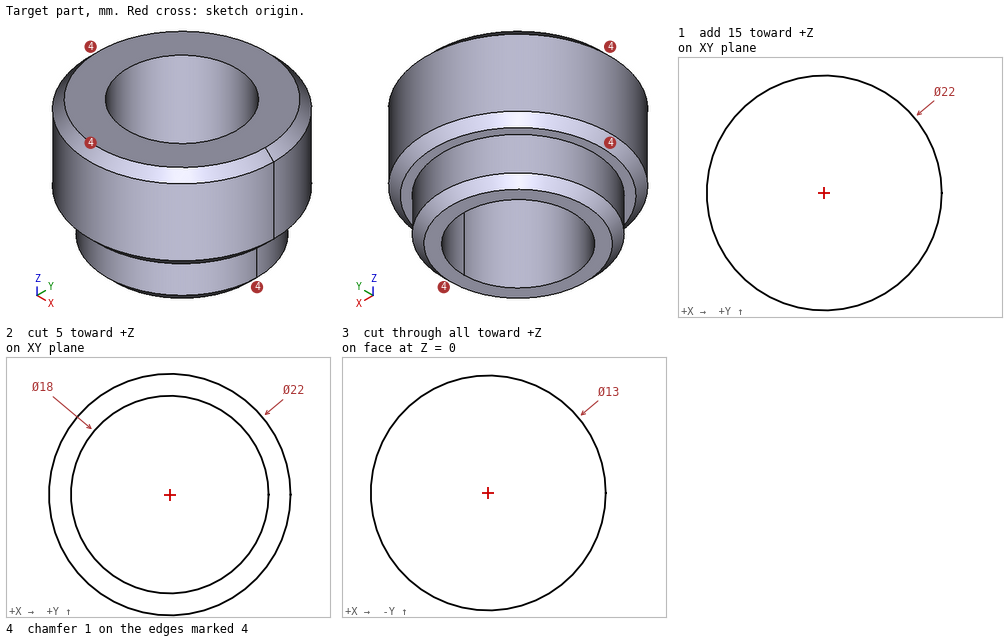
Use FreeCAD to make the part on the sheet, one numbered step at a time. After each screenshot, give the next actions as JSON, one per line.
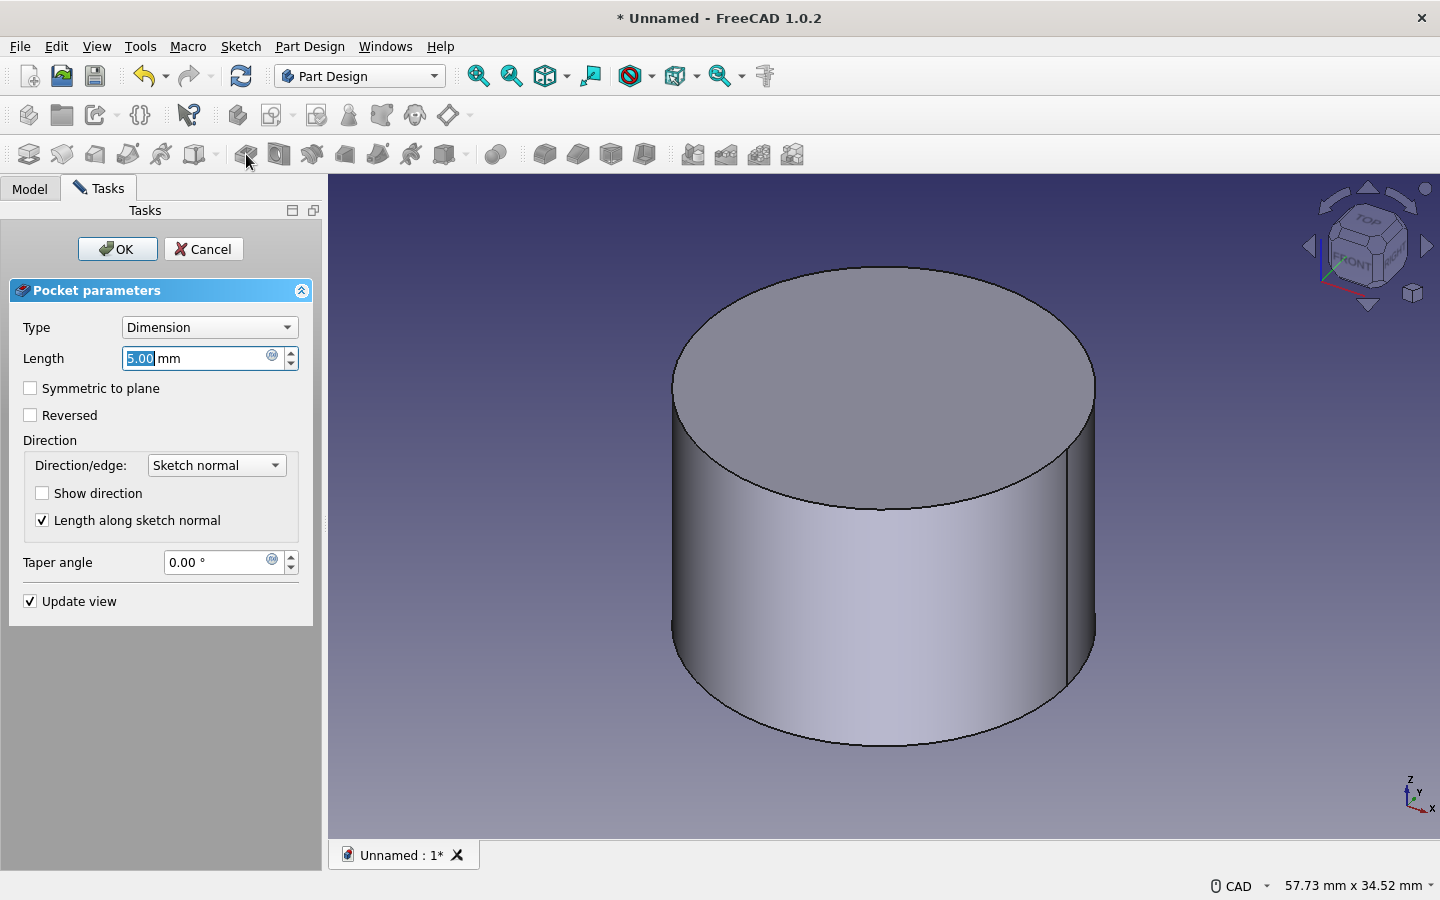
{"action": "type", "text": "5"}
{"action": "key", "text": "Tab"}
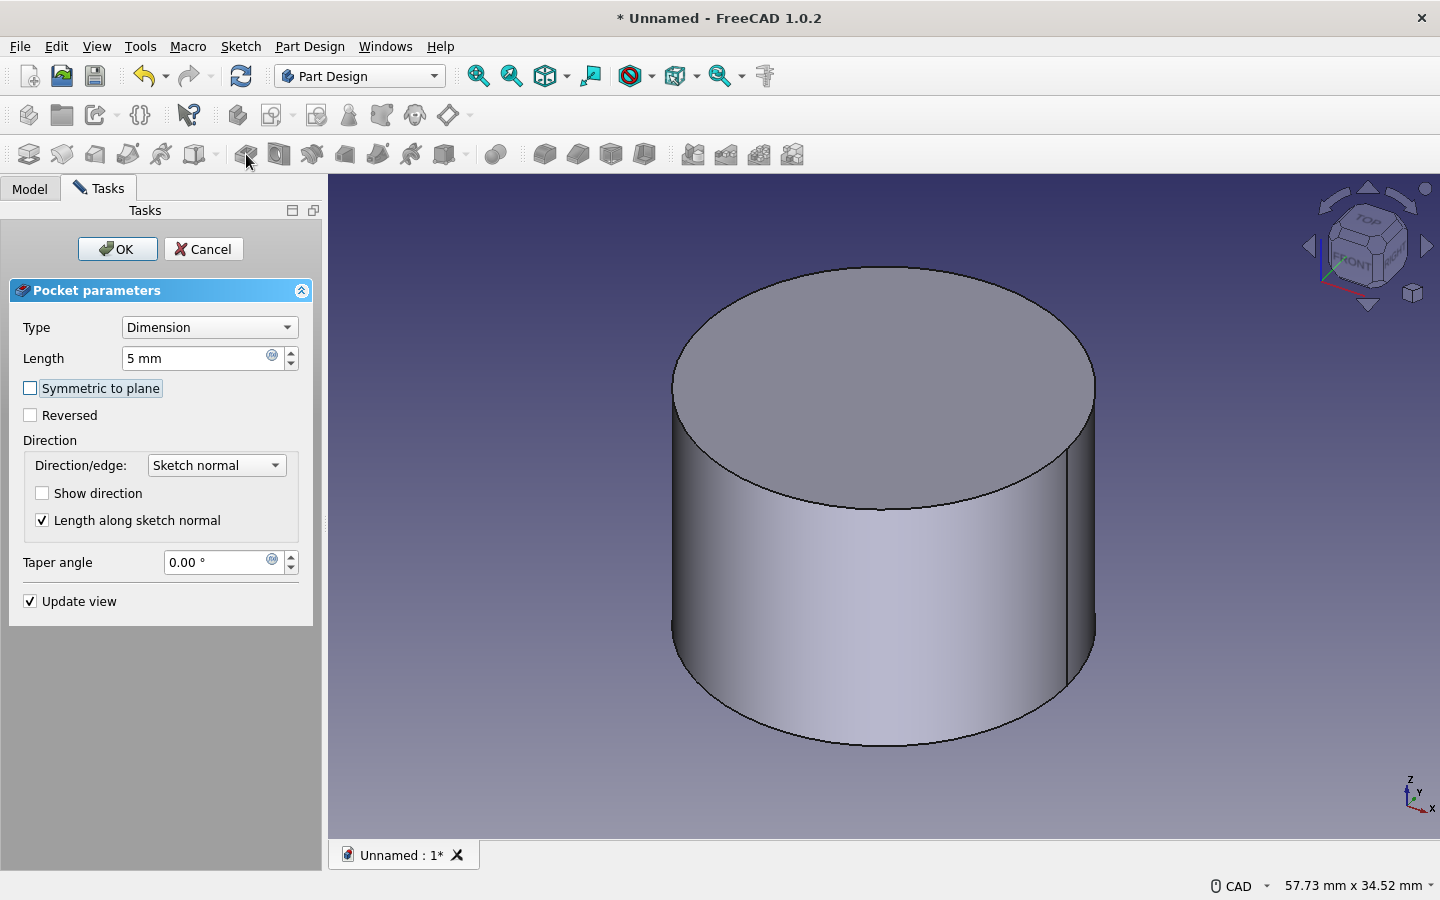
{"action": "left_click", "coordinate": [31, 415]}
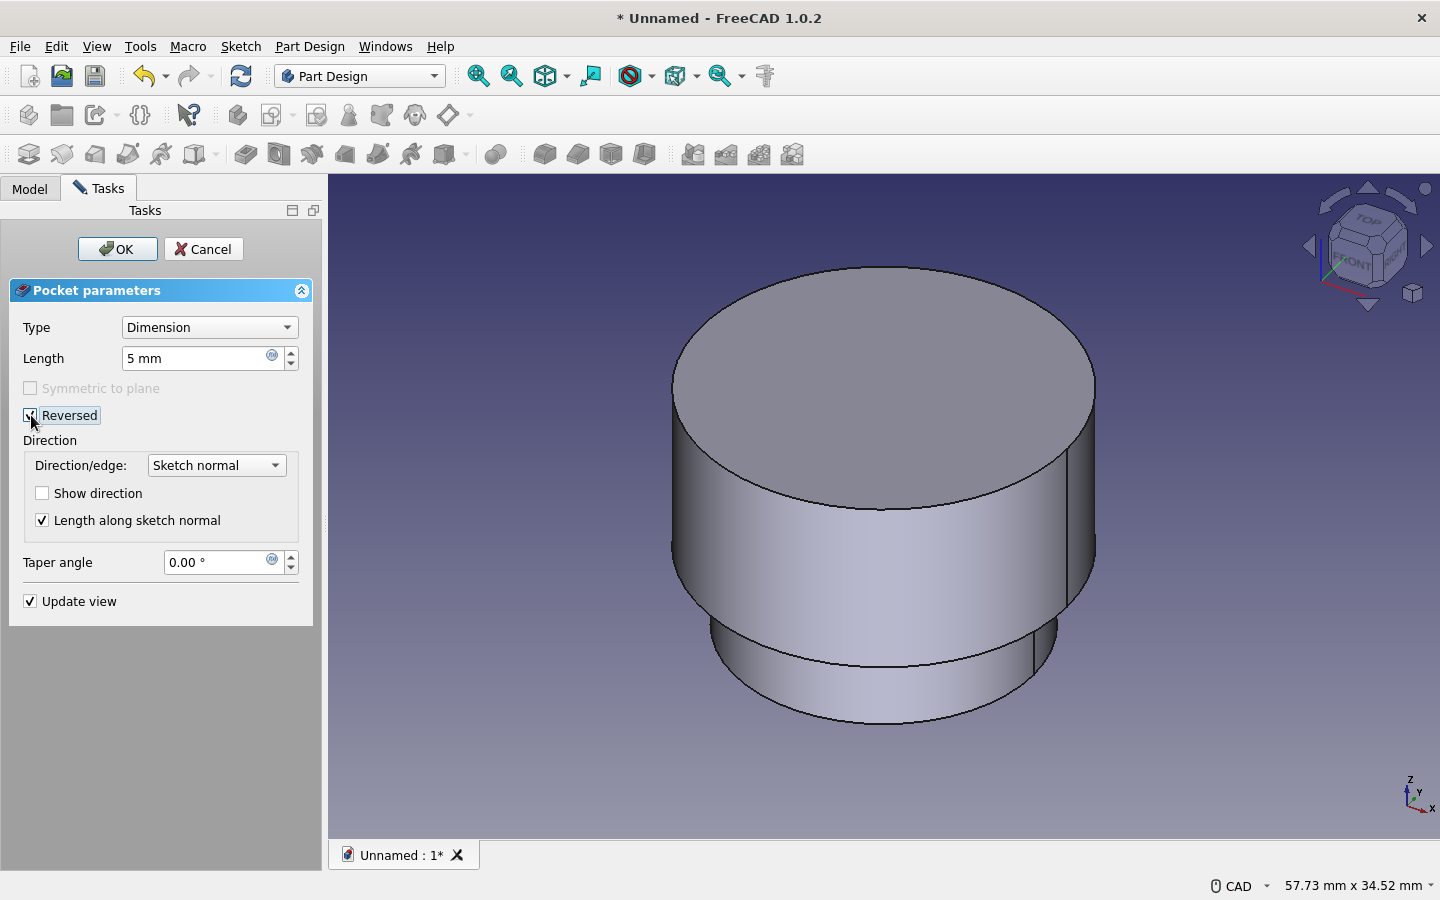
{"action": "left_click", "coordinate": [118, 249]}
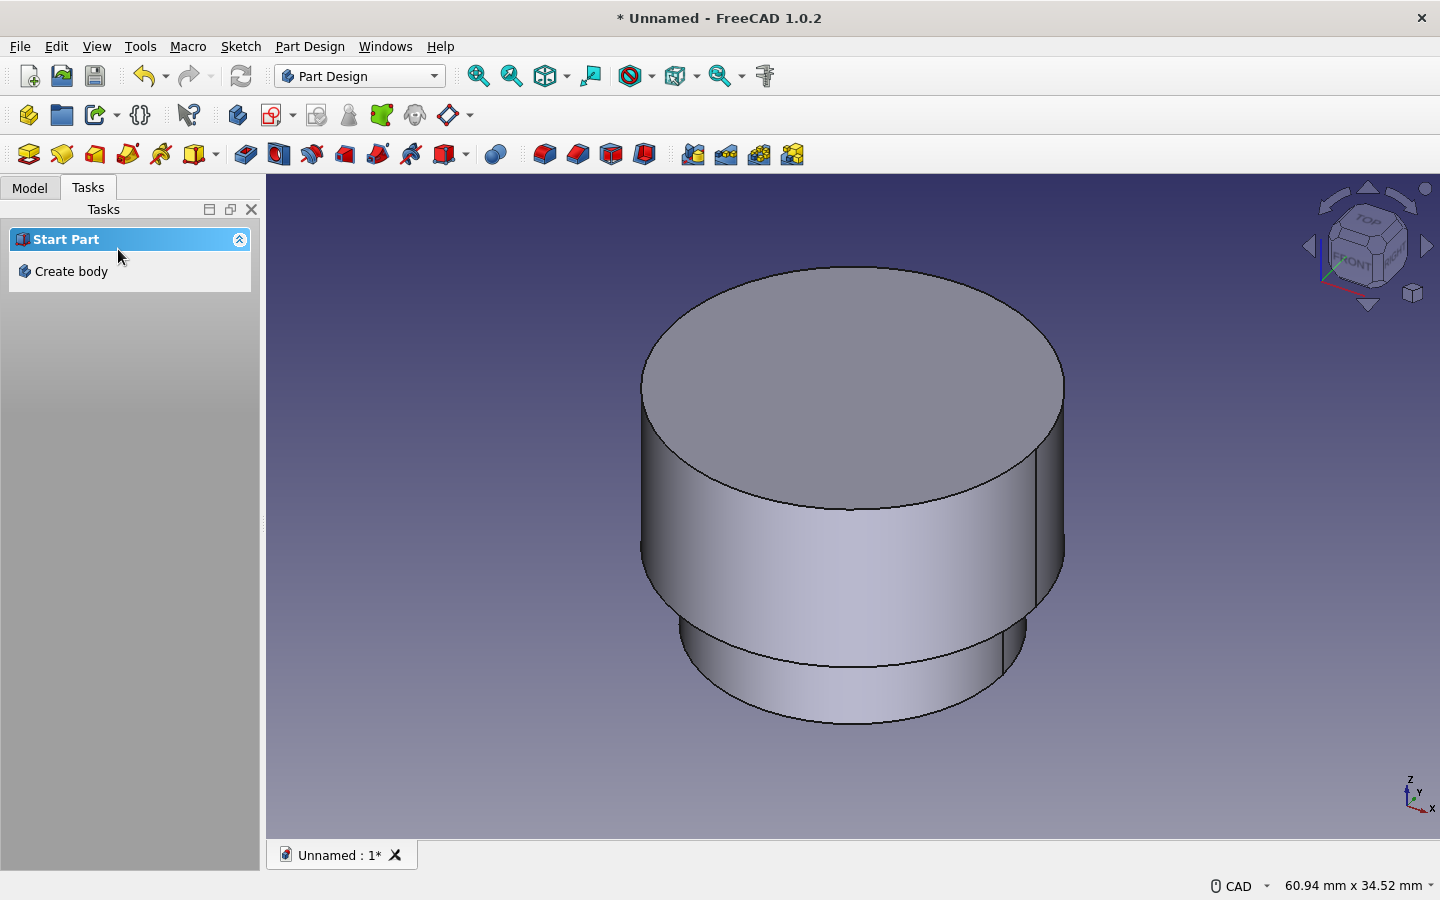
{"action": "key", "text": "5"}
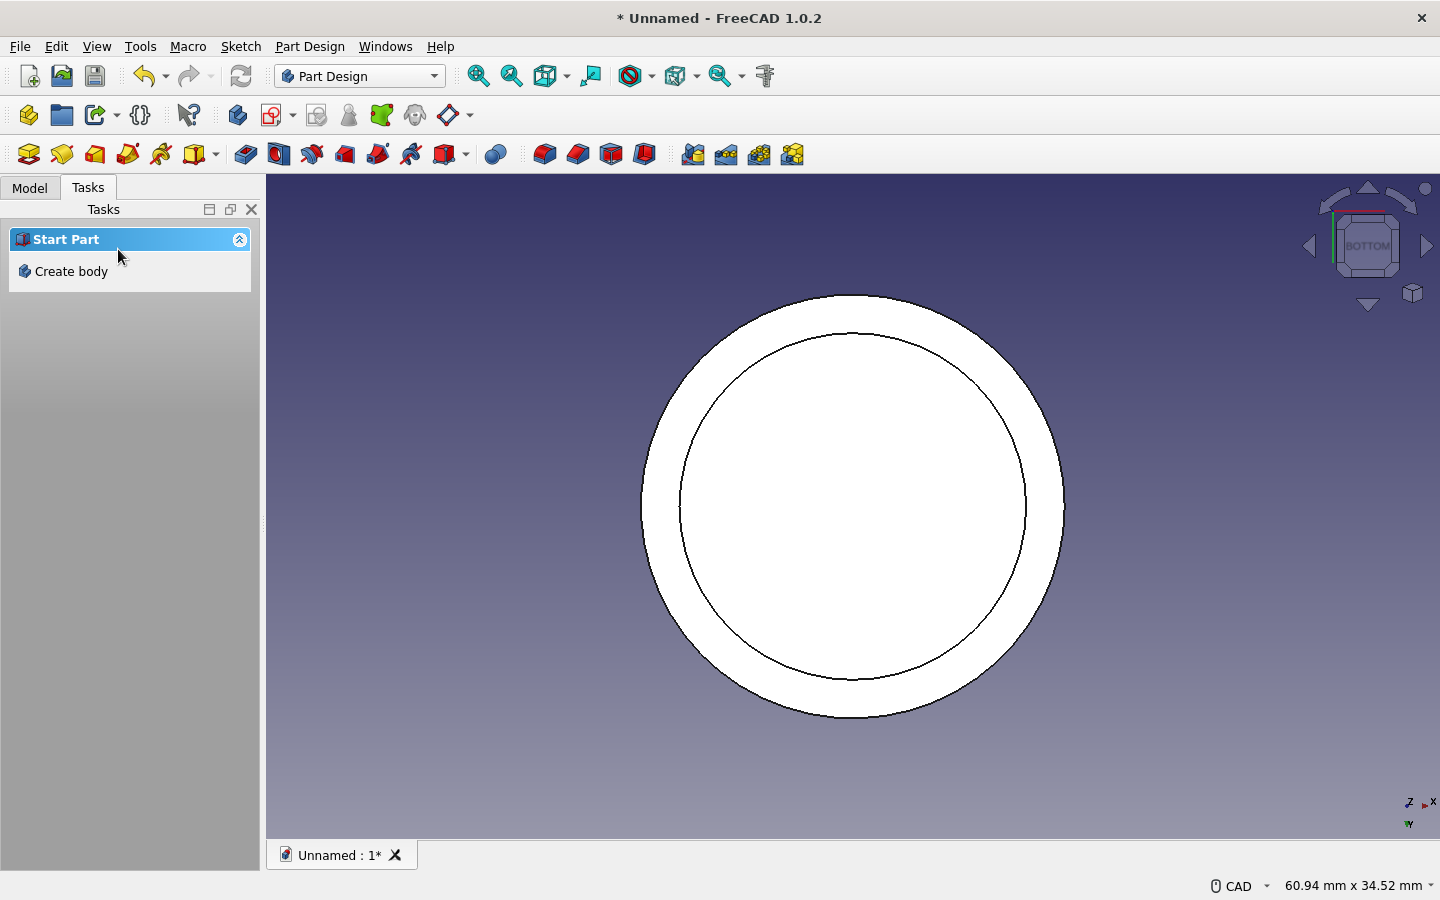
{"action": "left_click", "coordinate": [853, 505]}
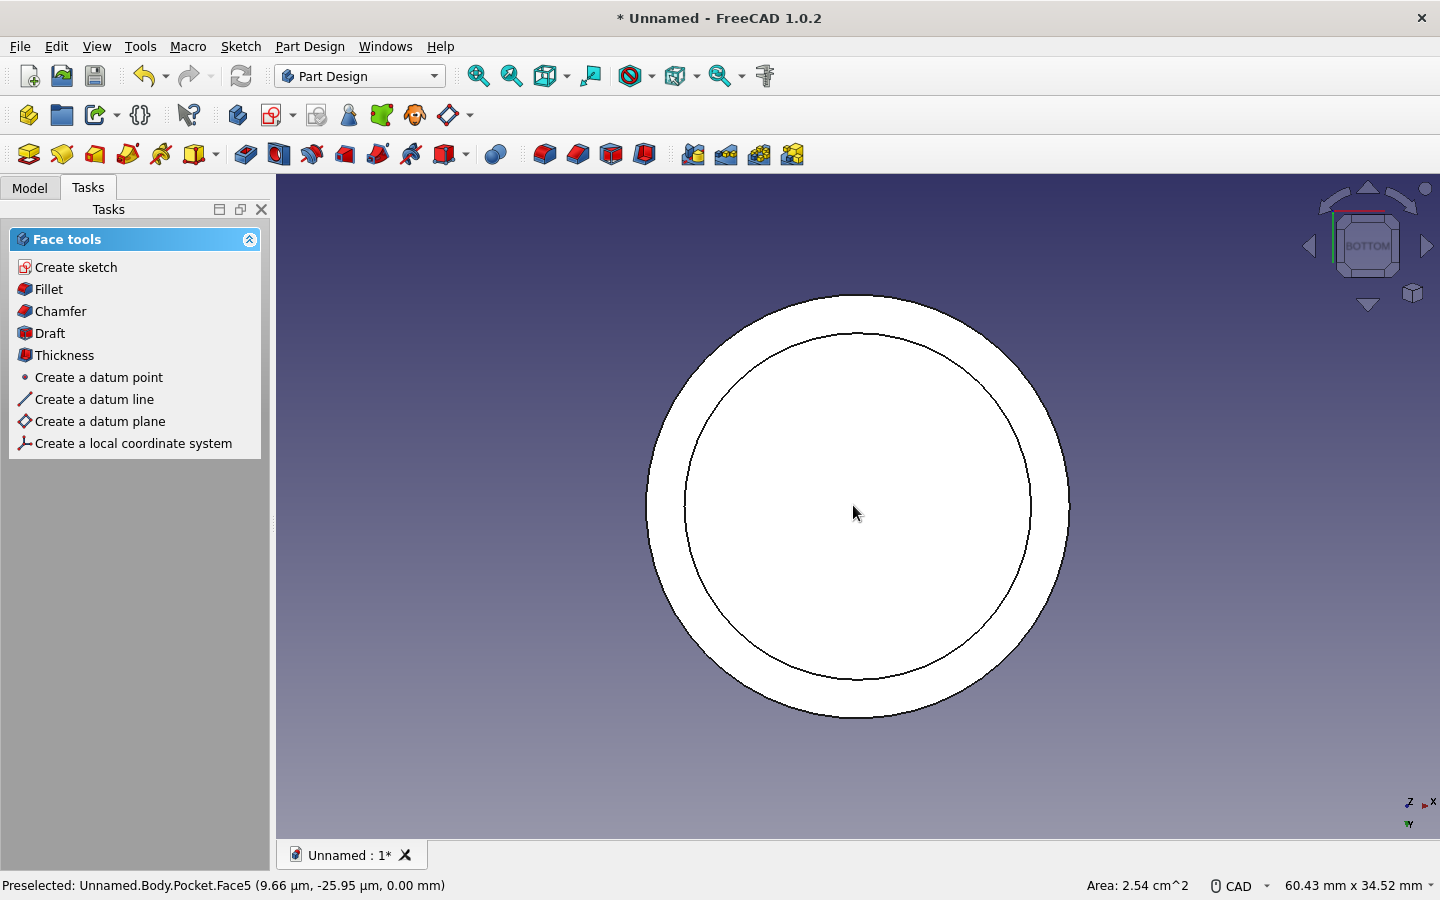
{"action": "left_click", "coordinate": [270, 116]}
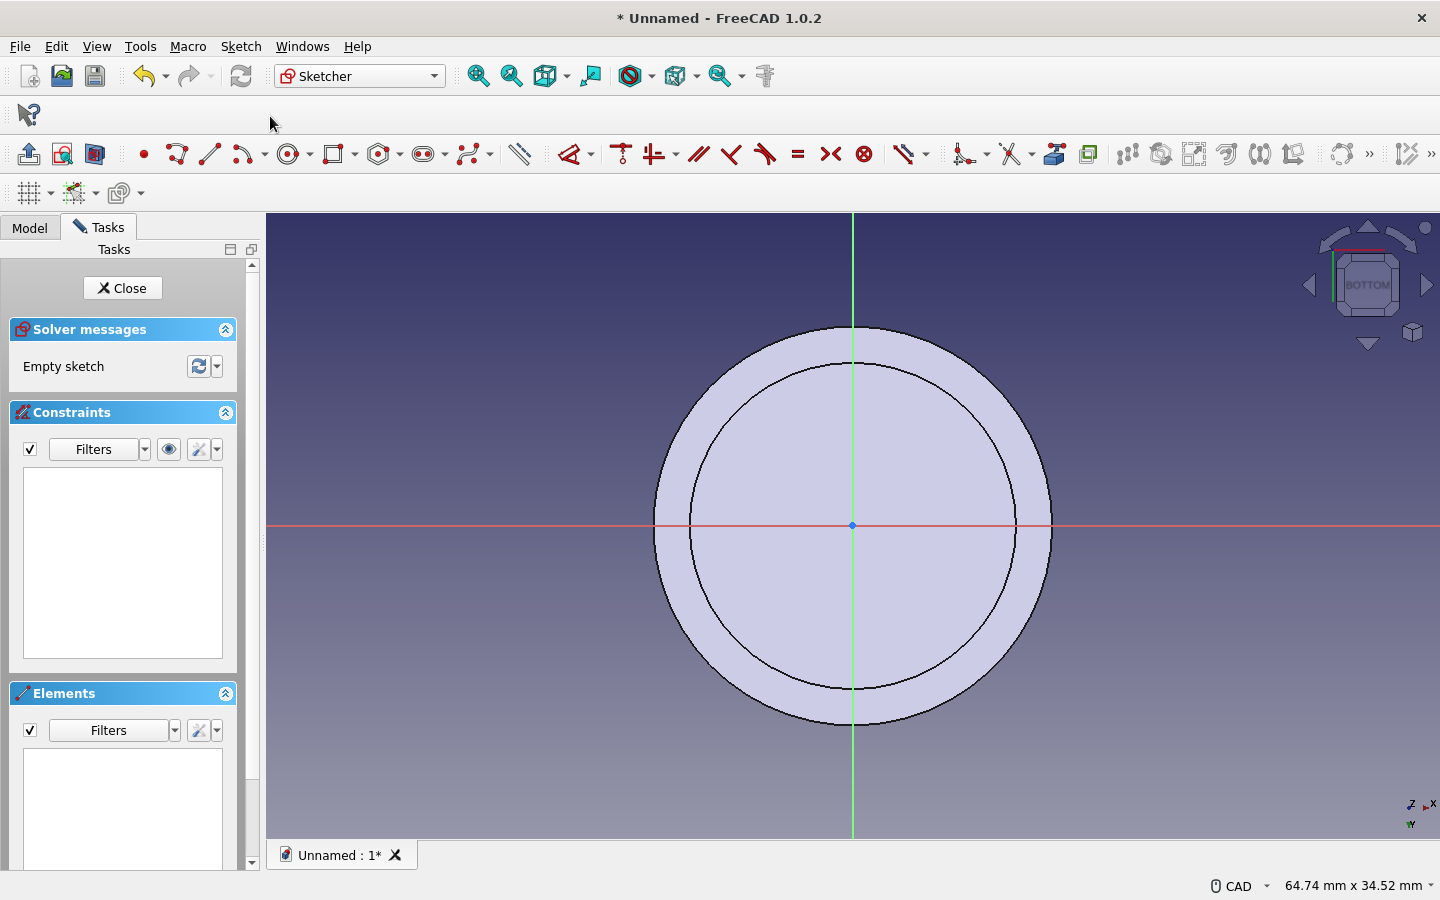
{"action": "scroll", "coordinate": [936, 526], "scroll_direction": "up", "scroll_amount": 3}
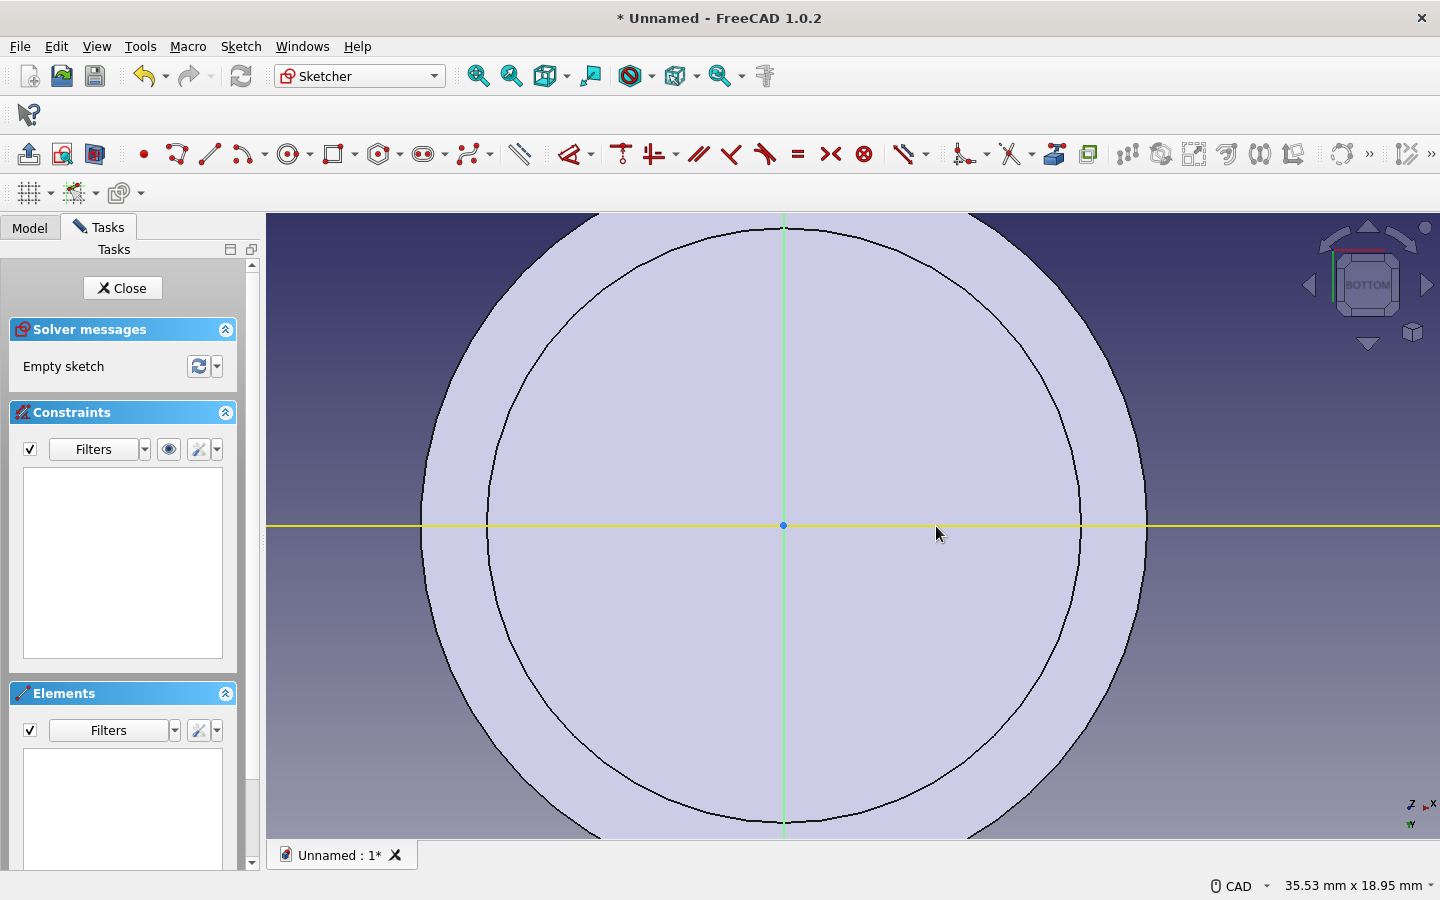
{"action": "left_click", "coordinate": [288, 154]}